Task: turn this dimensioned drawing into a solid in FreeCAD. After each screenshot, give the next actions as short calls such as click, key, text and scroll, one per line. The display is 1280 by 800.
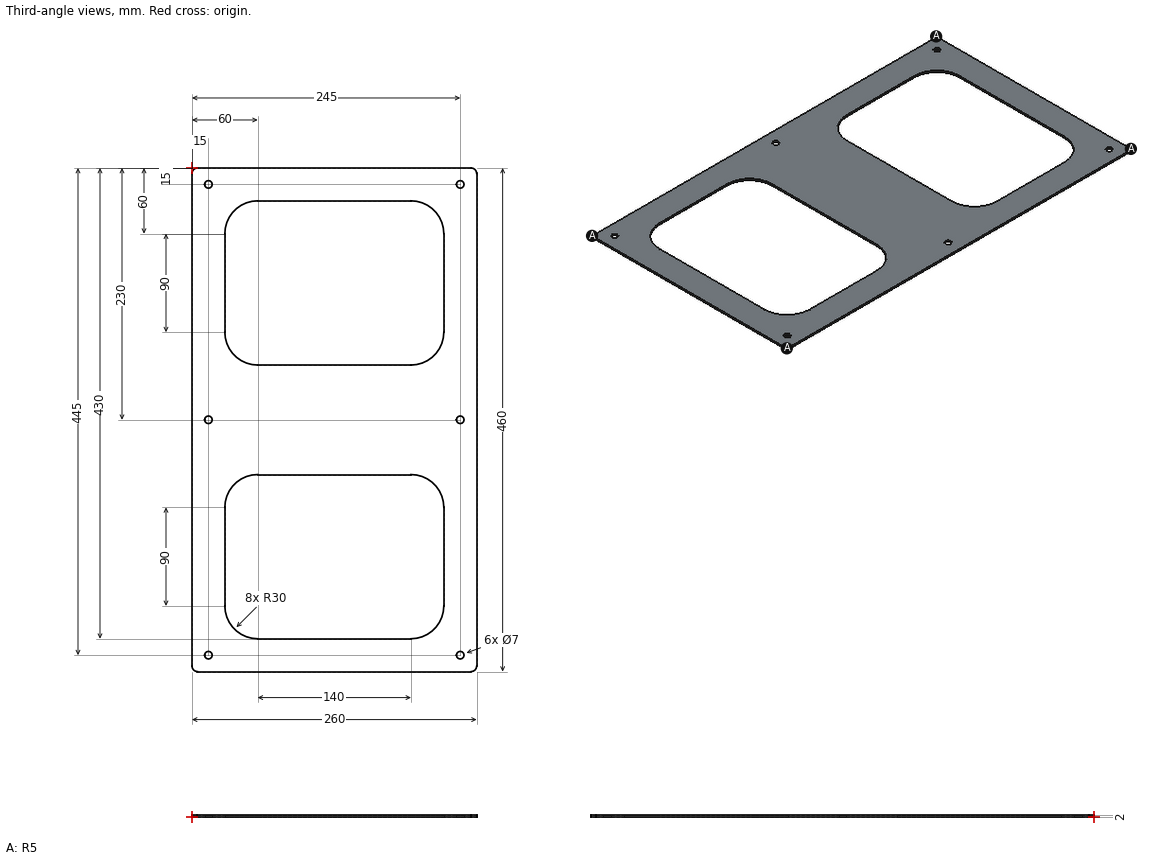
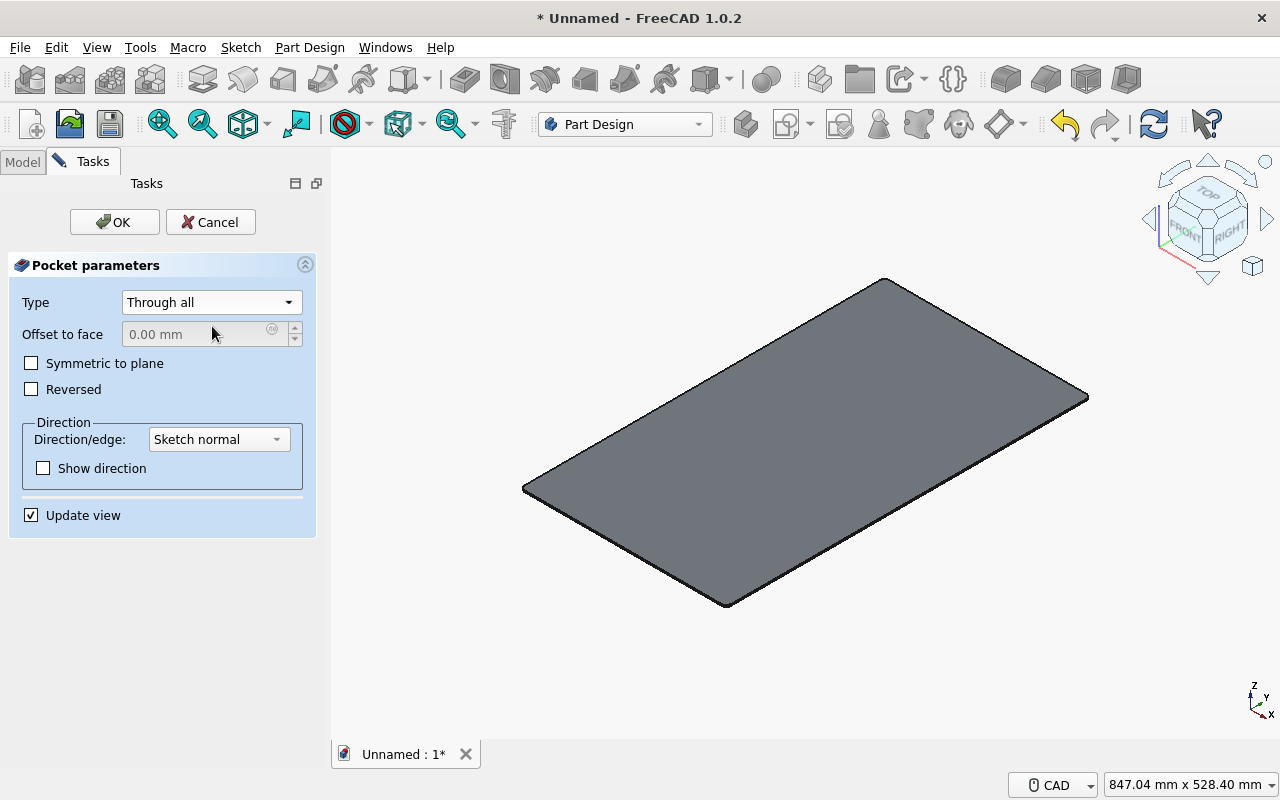
click(30, 389)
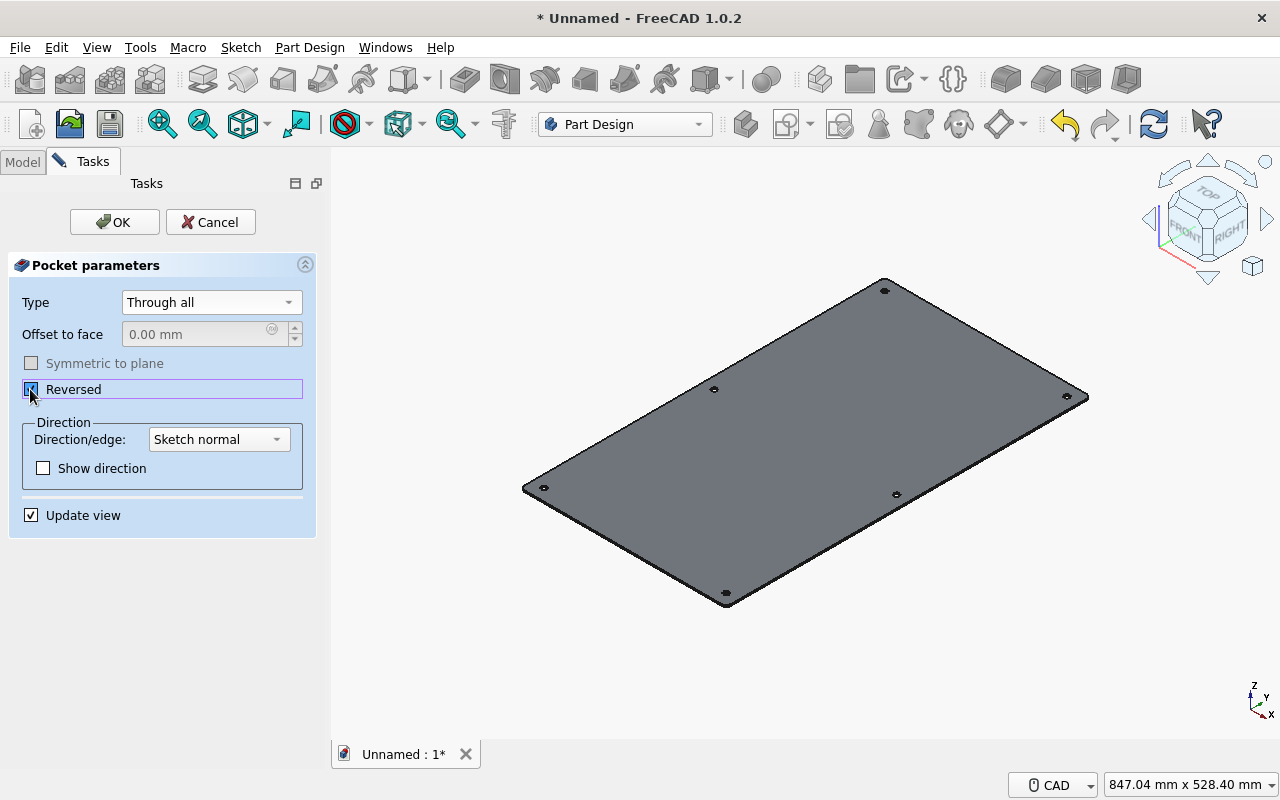
click(115, 222)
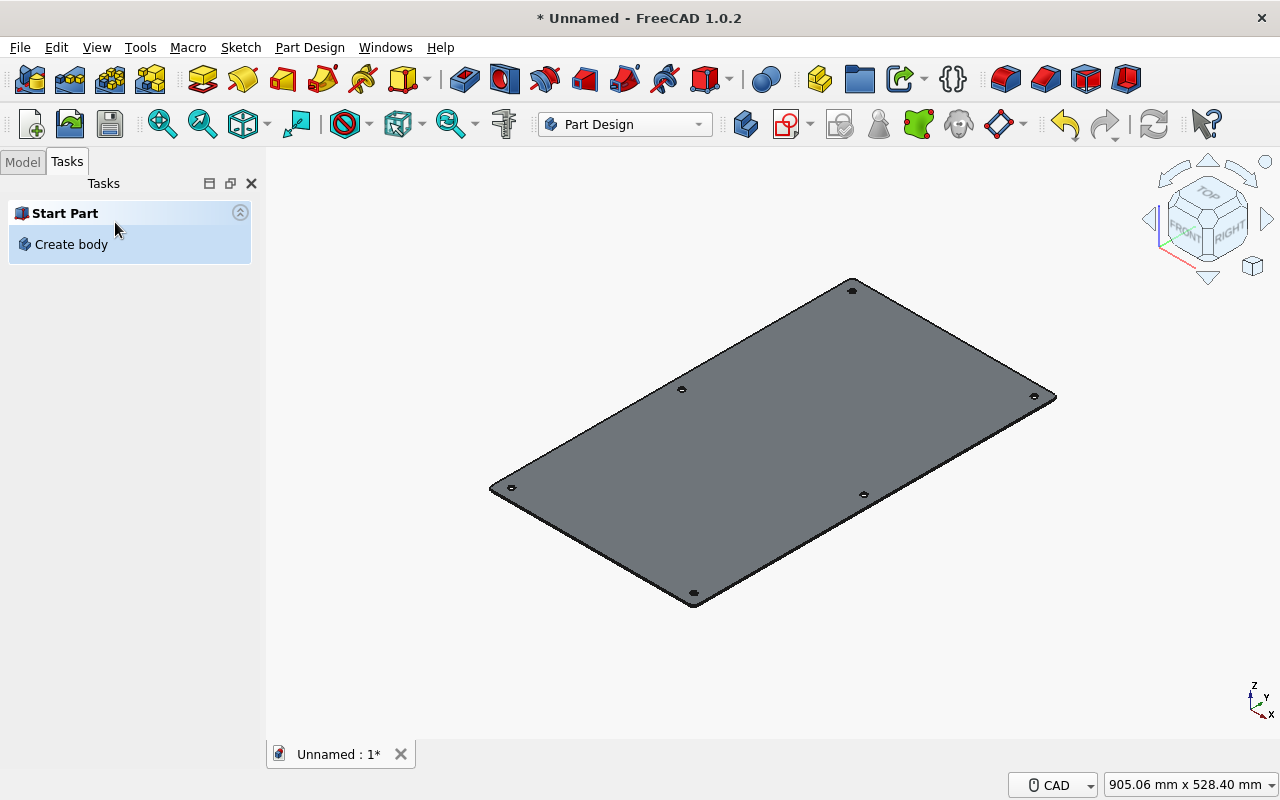
key(5)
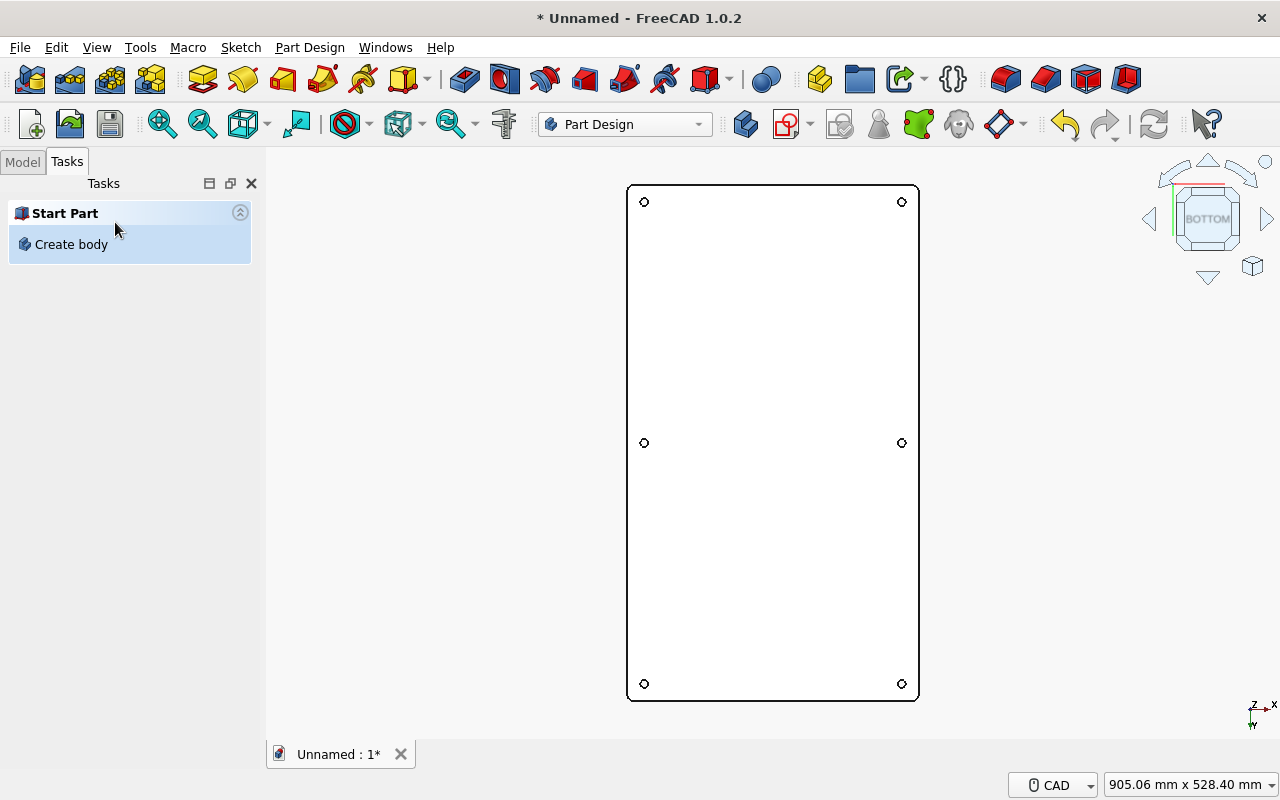
click(773, 516)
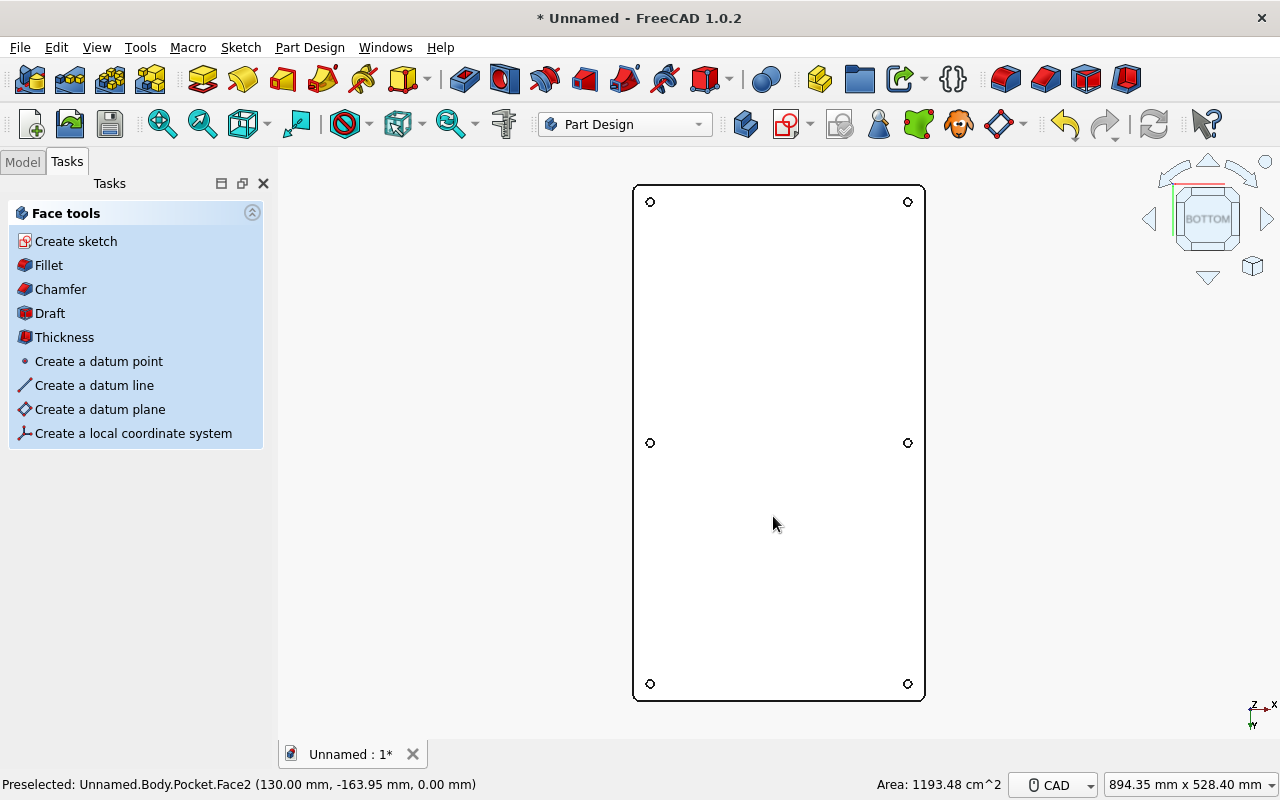
click(786, 124)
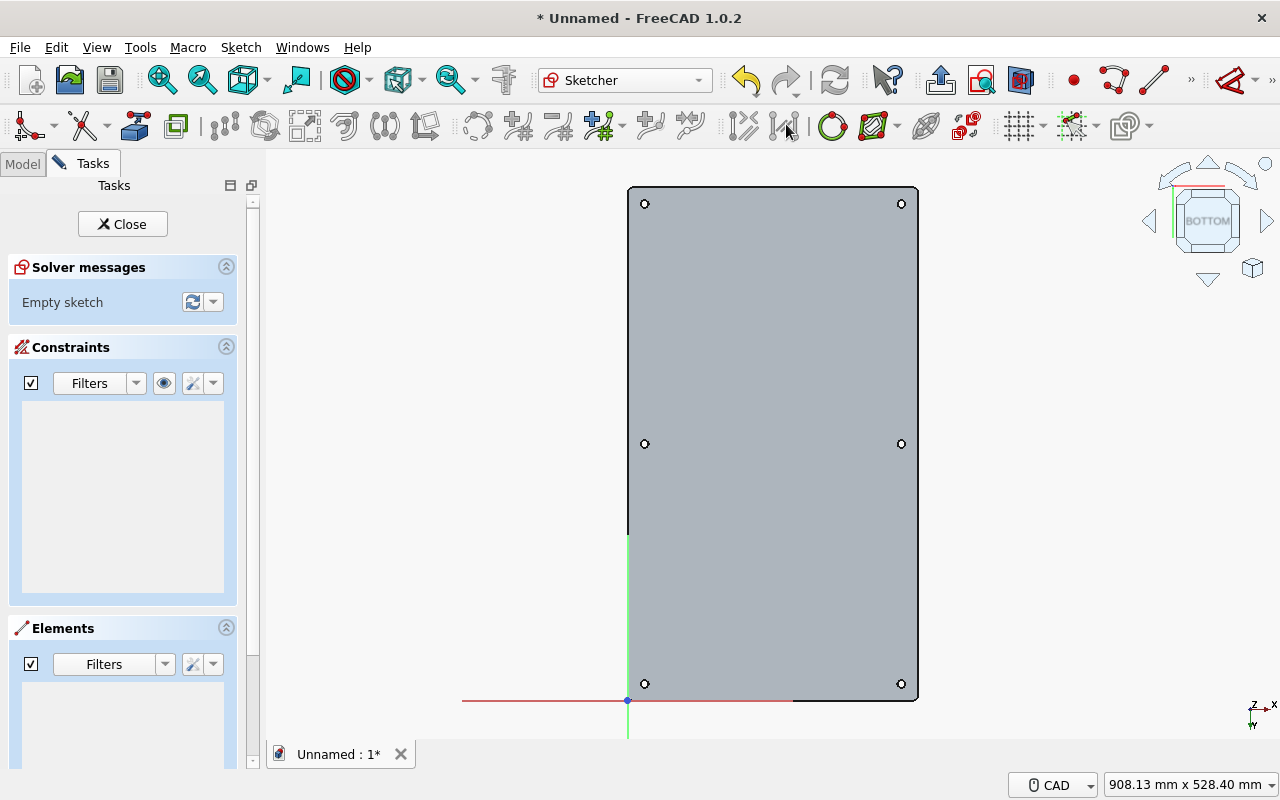
scroll(471, 368, down, 1)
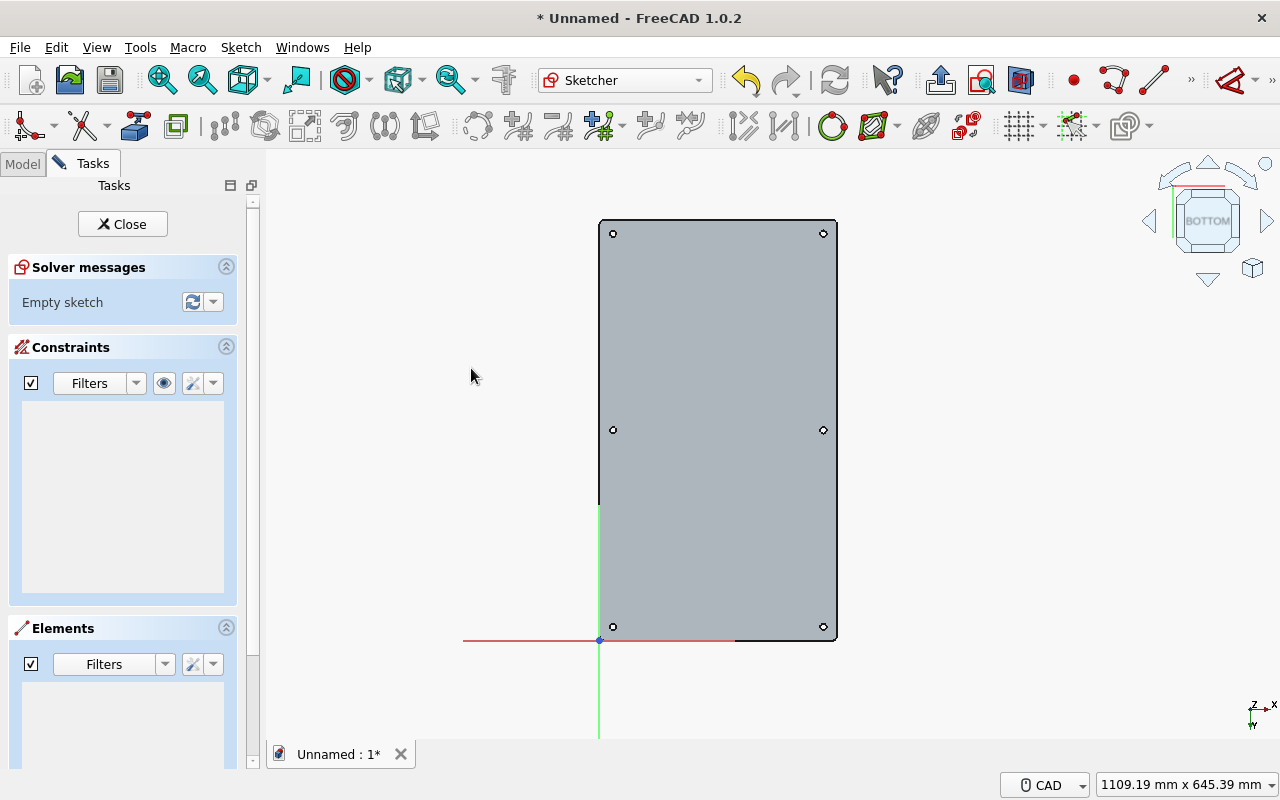
click(1154, 80)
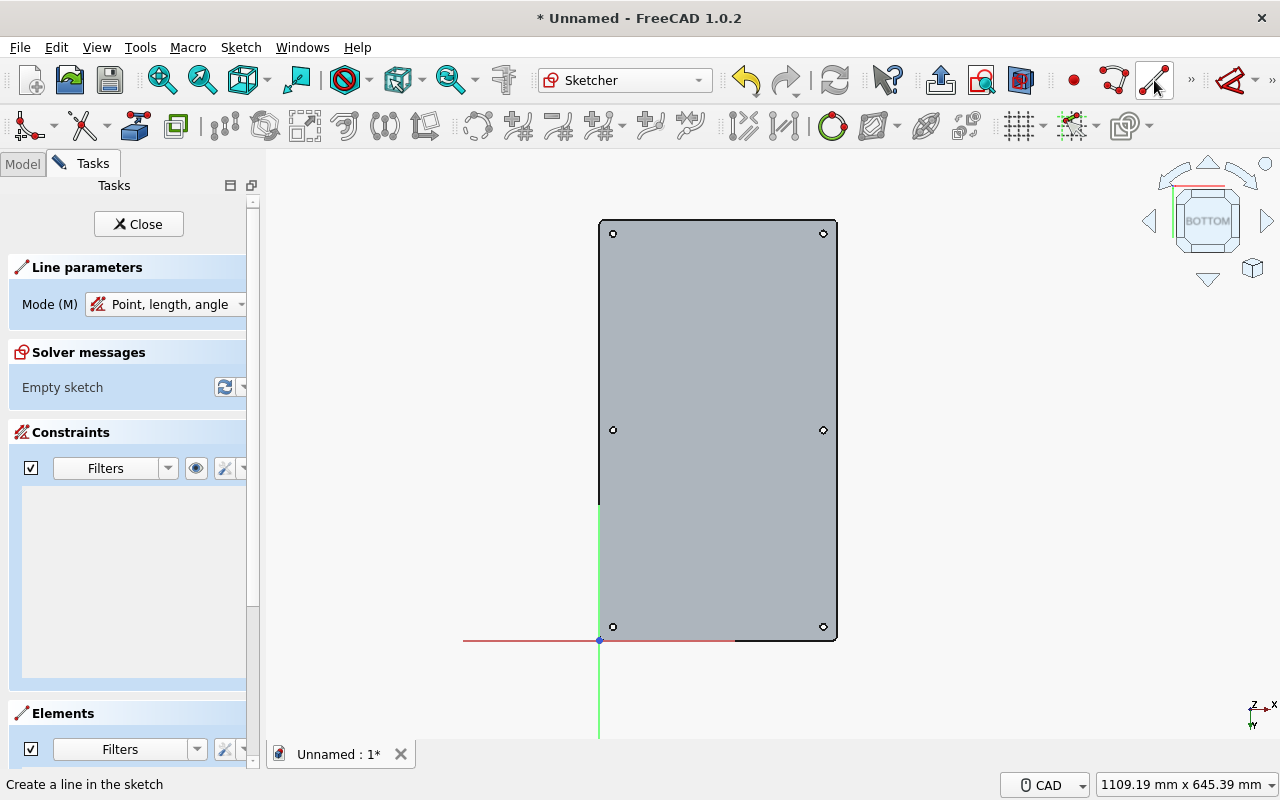
click(782, 247)
click(654, 247)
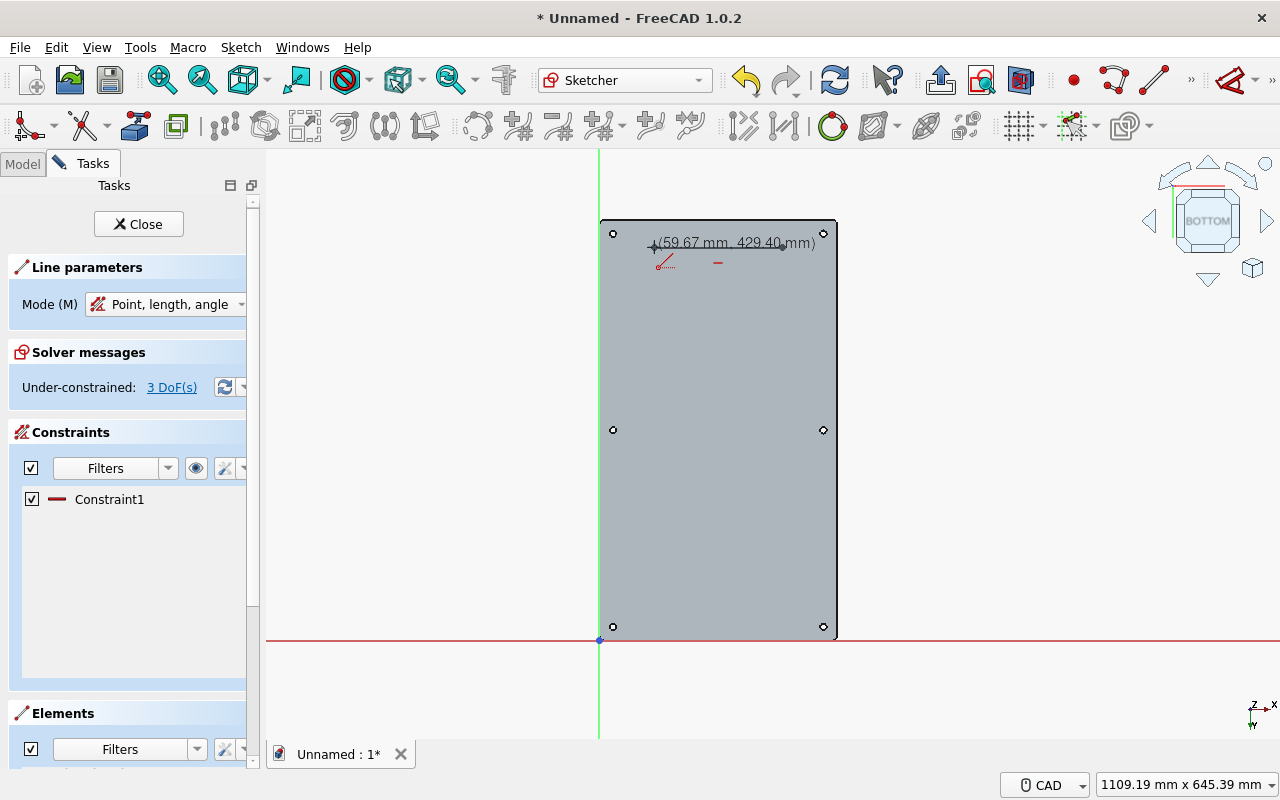
click(627, 275)
click(627, 357)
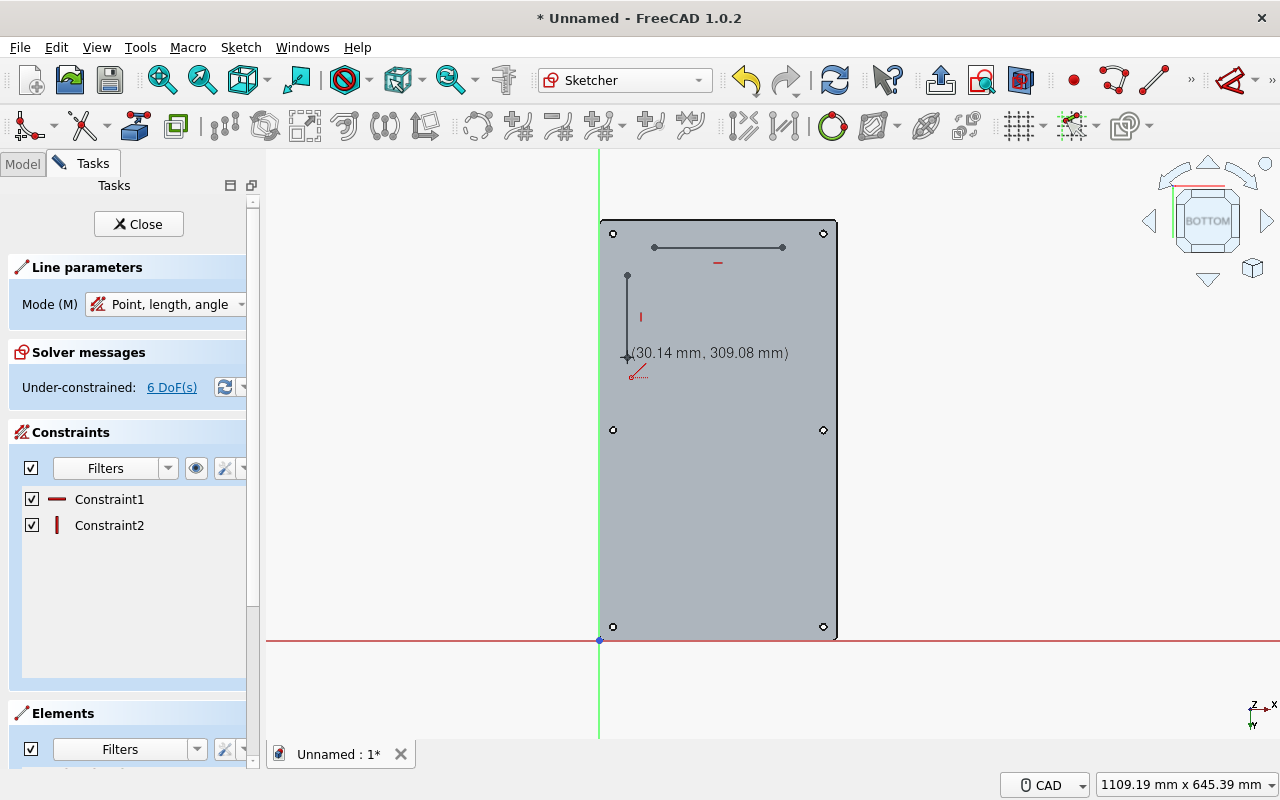
click(654, 385)
click(782, 385)